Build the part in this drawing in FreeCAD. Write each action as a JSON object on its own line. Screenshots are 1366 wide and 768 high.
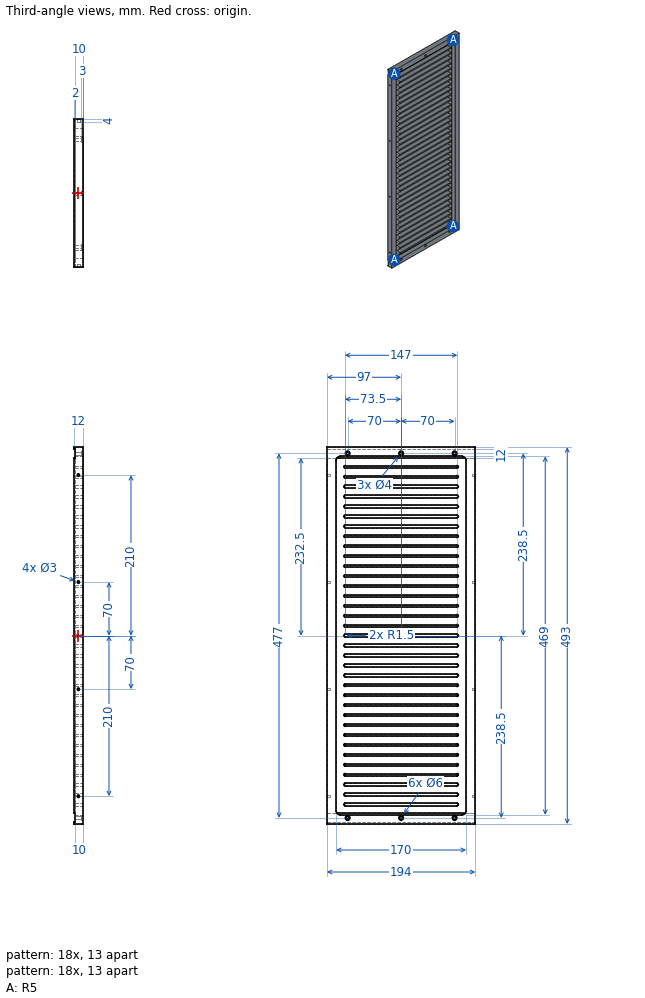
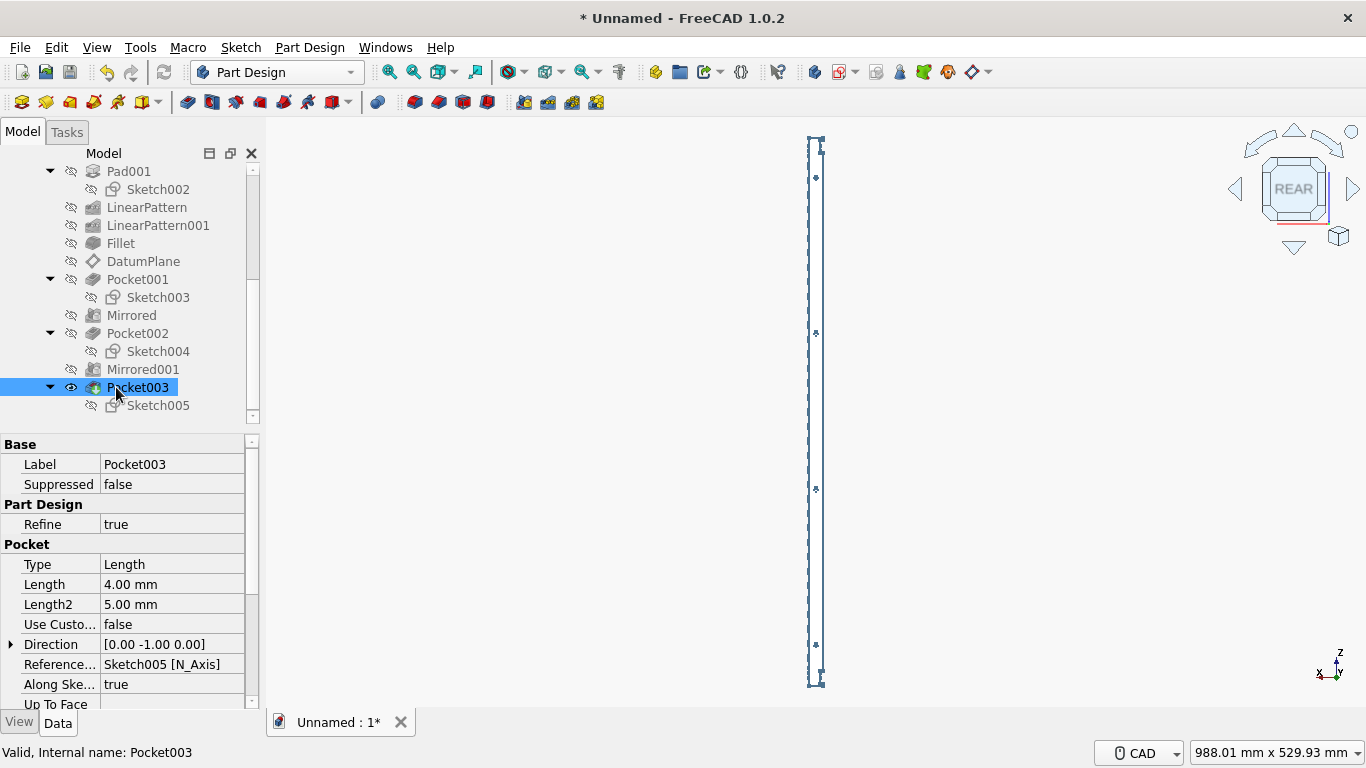
{"action": "left_click", "coordinate": [524, 102]}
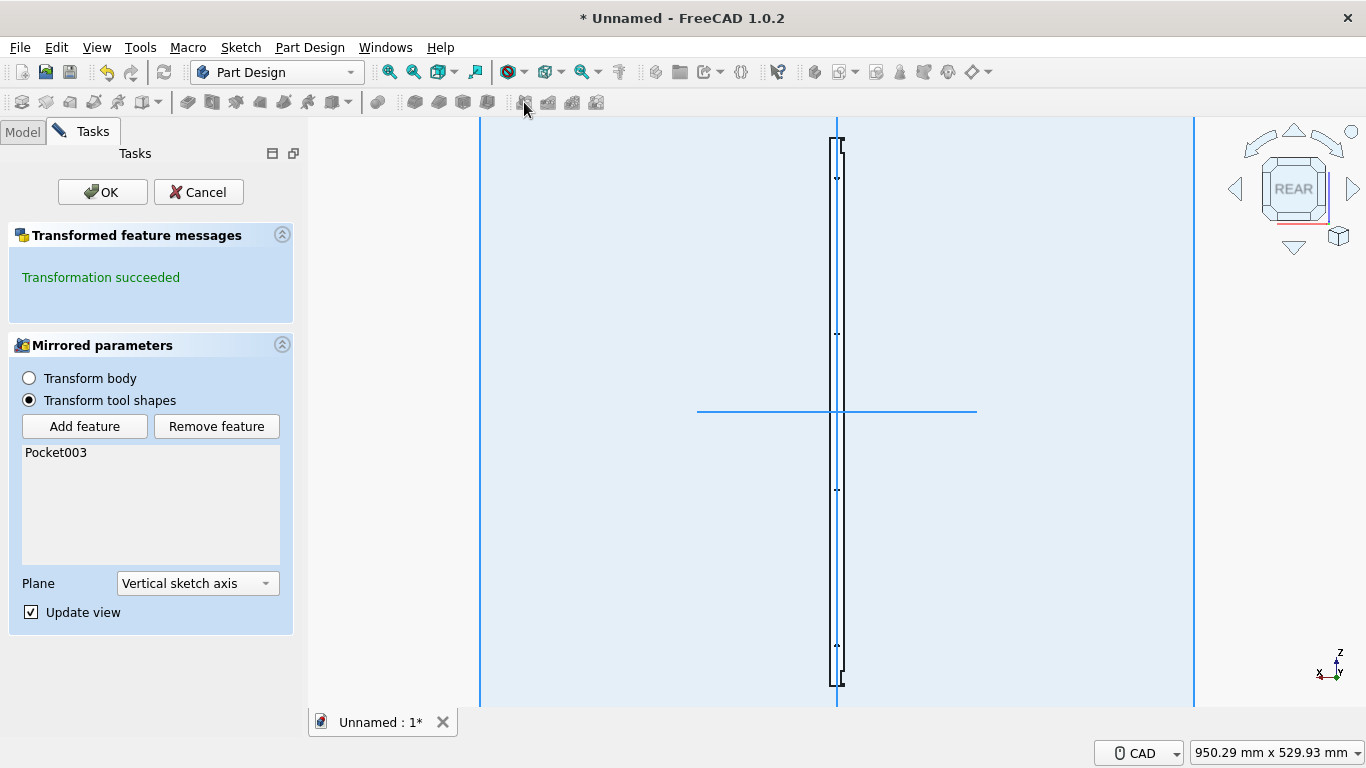
{"action": "left_click", "coordinate": [198, 584]}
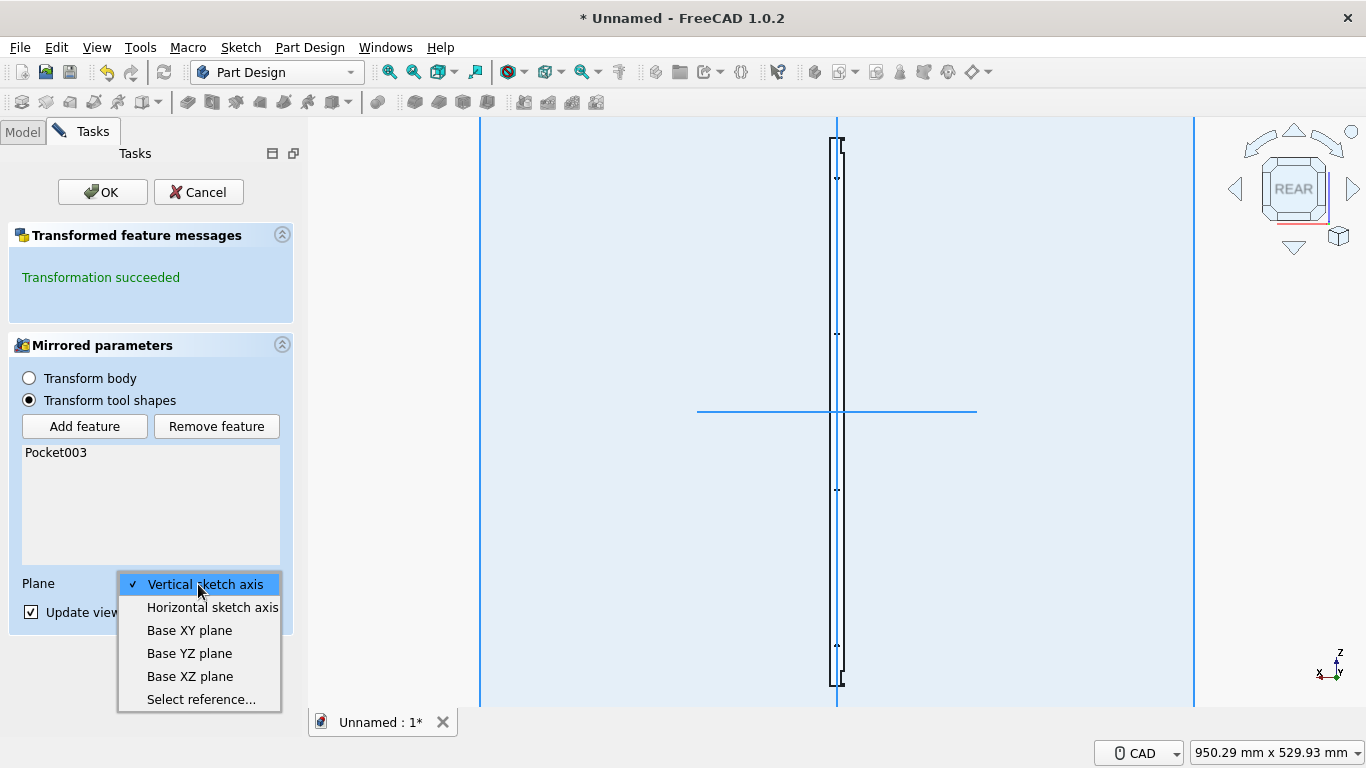
{"action": "left_click", "coordinate": [198, 676]}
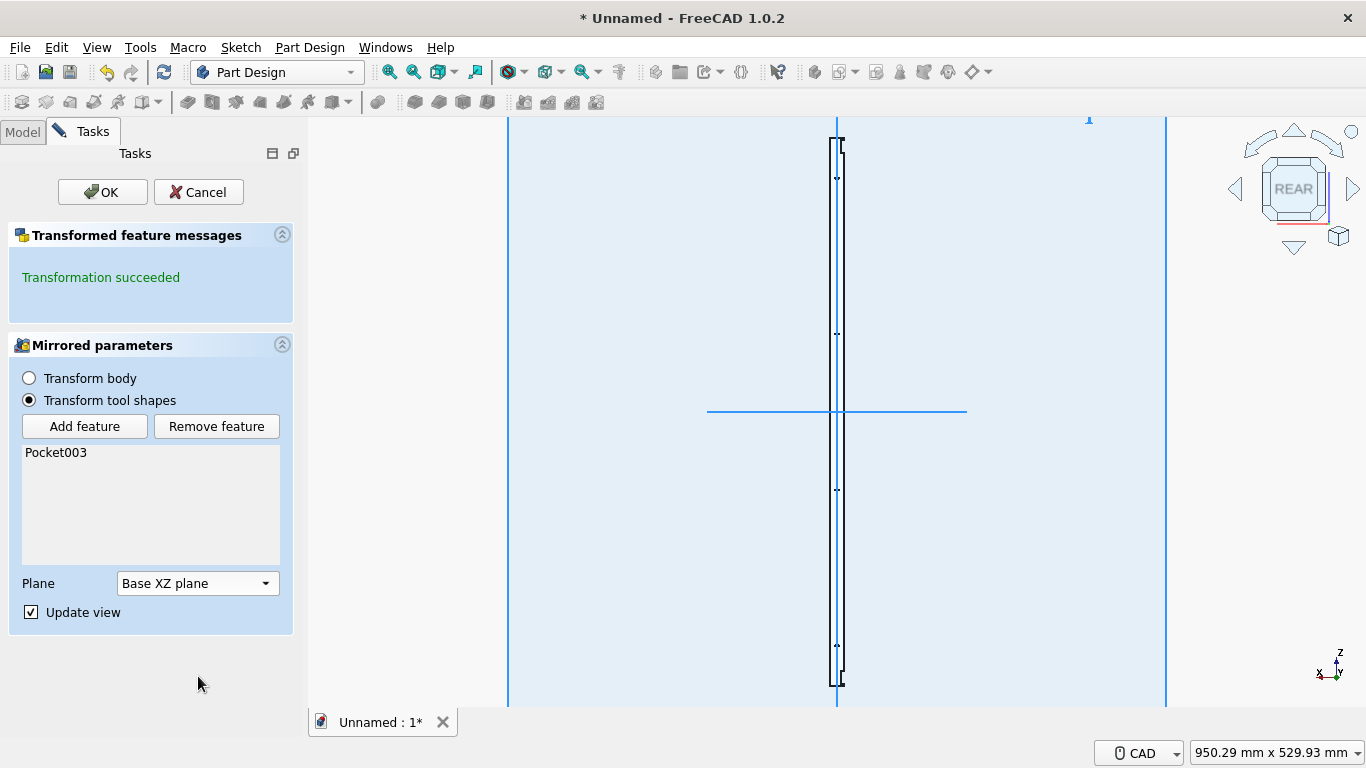
{"action": "left_click", "coordinate": [103, 192]}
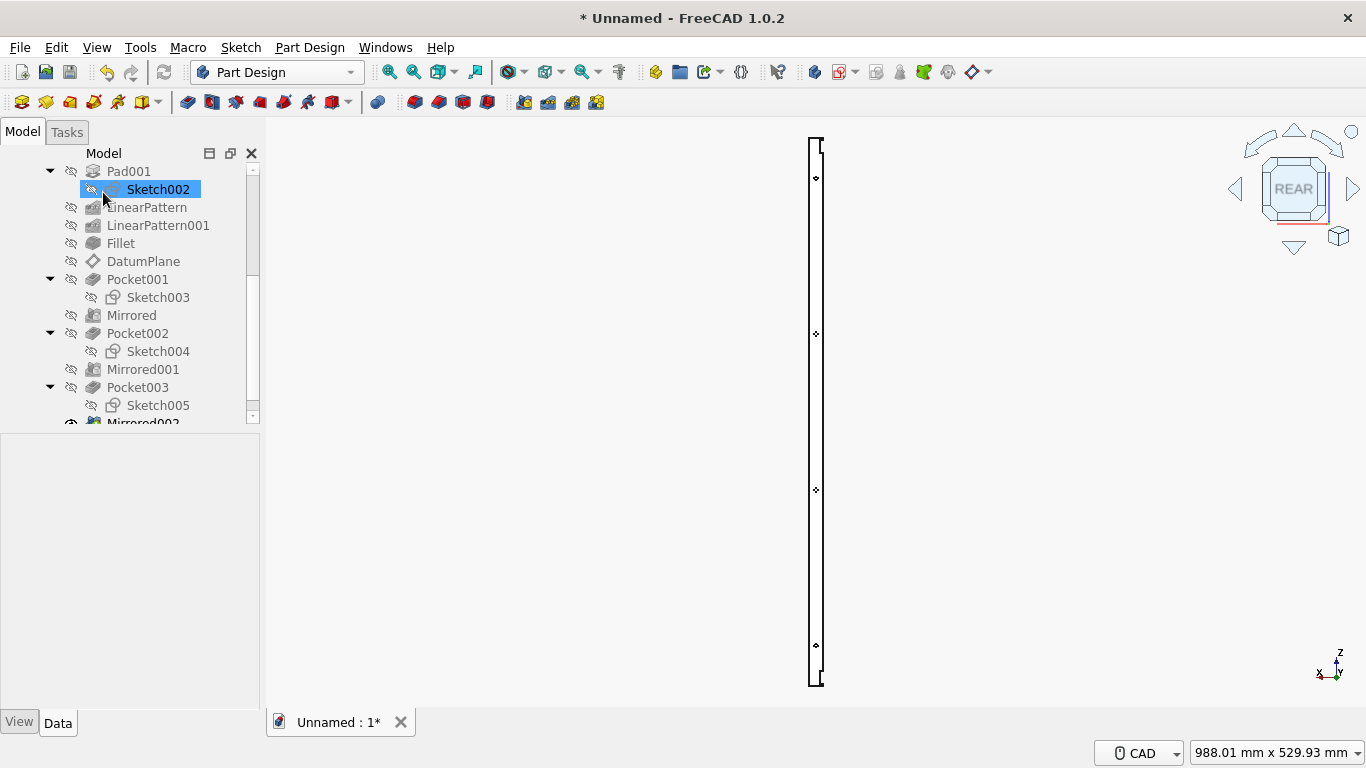
{"action": "key", "text": "0"}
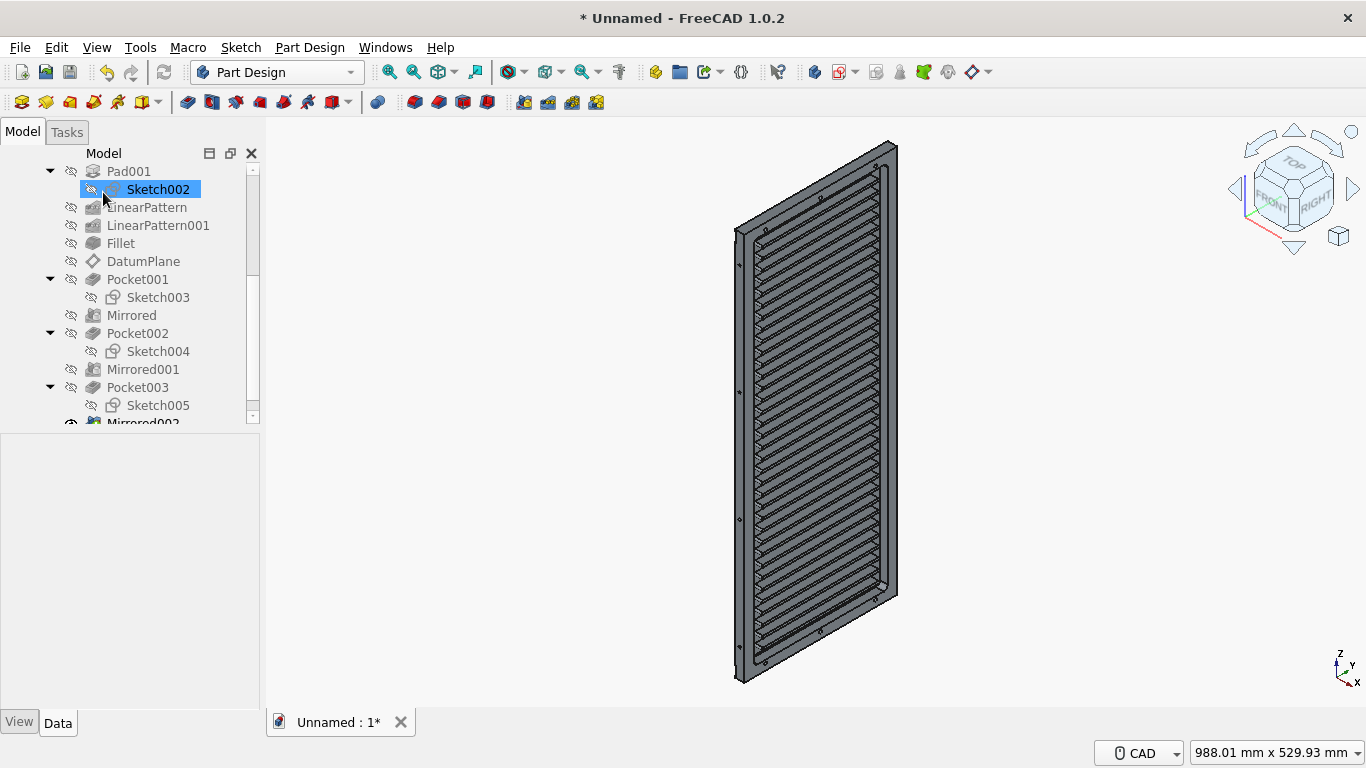
{"action": "key", "text": "3"}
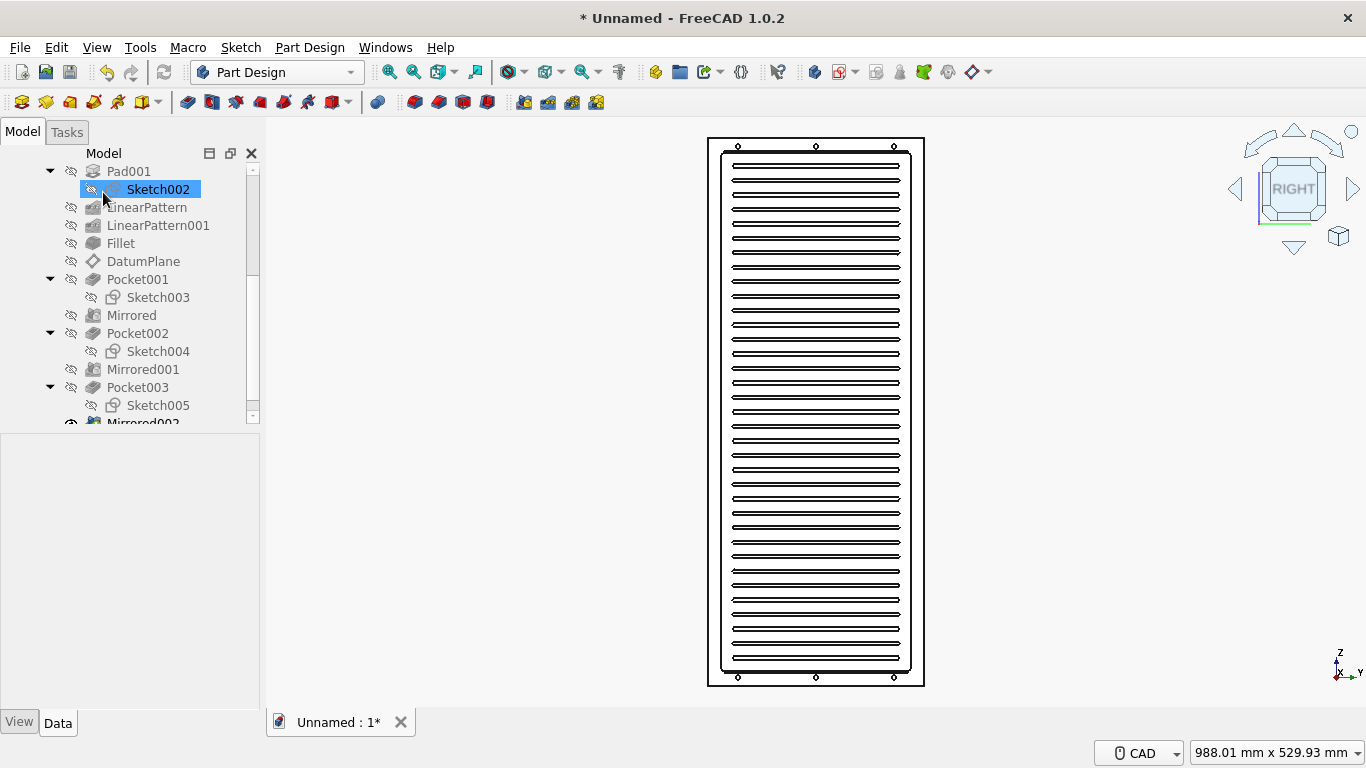
{"action": "key", "text": "2"}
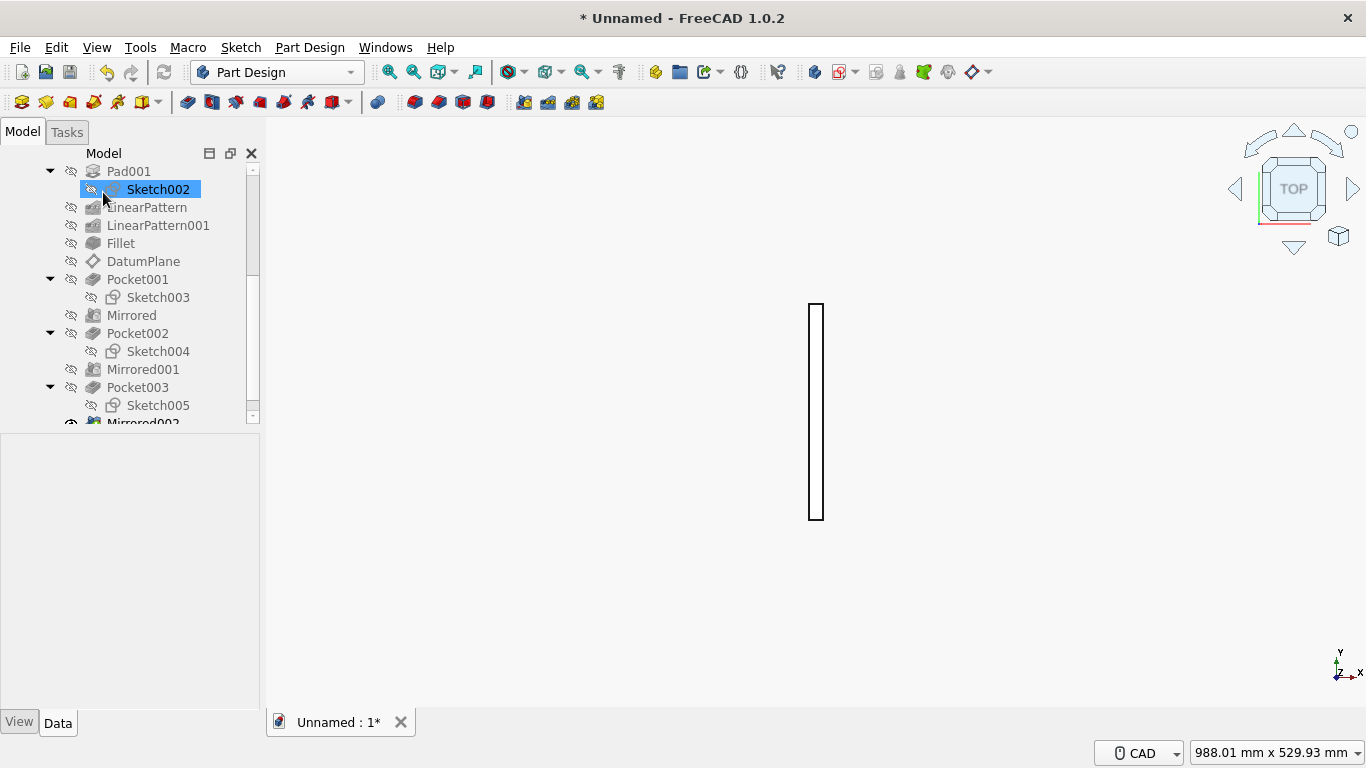
{"action": "left_click", "coordinate": [390, 72]}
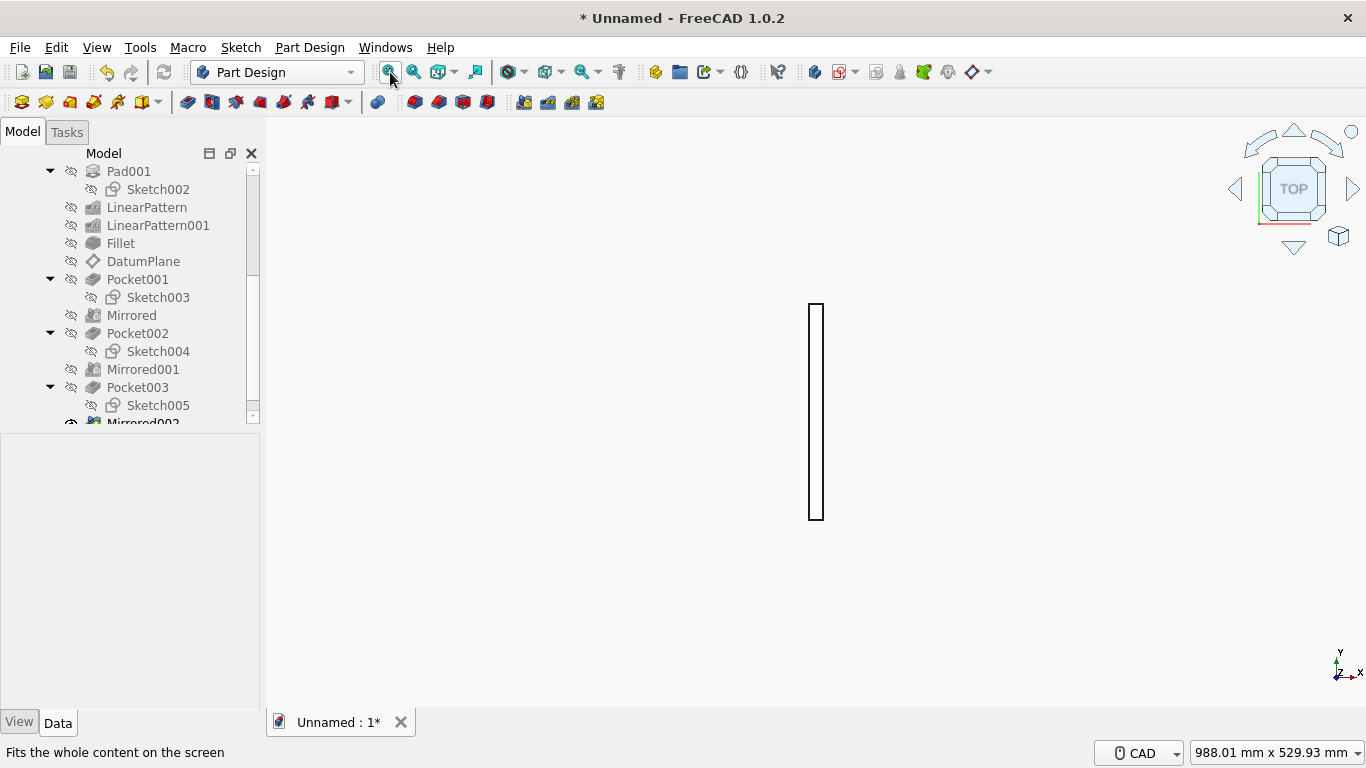
{"action": "scroll", "coordinate": [140, 293], "scroll_direction": "down", "scroll_amount": 3}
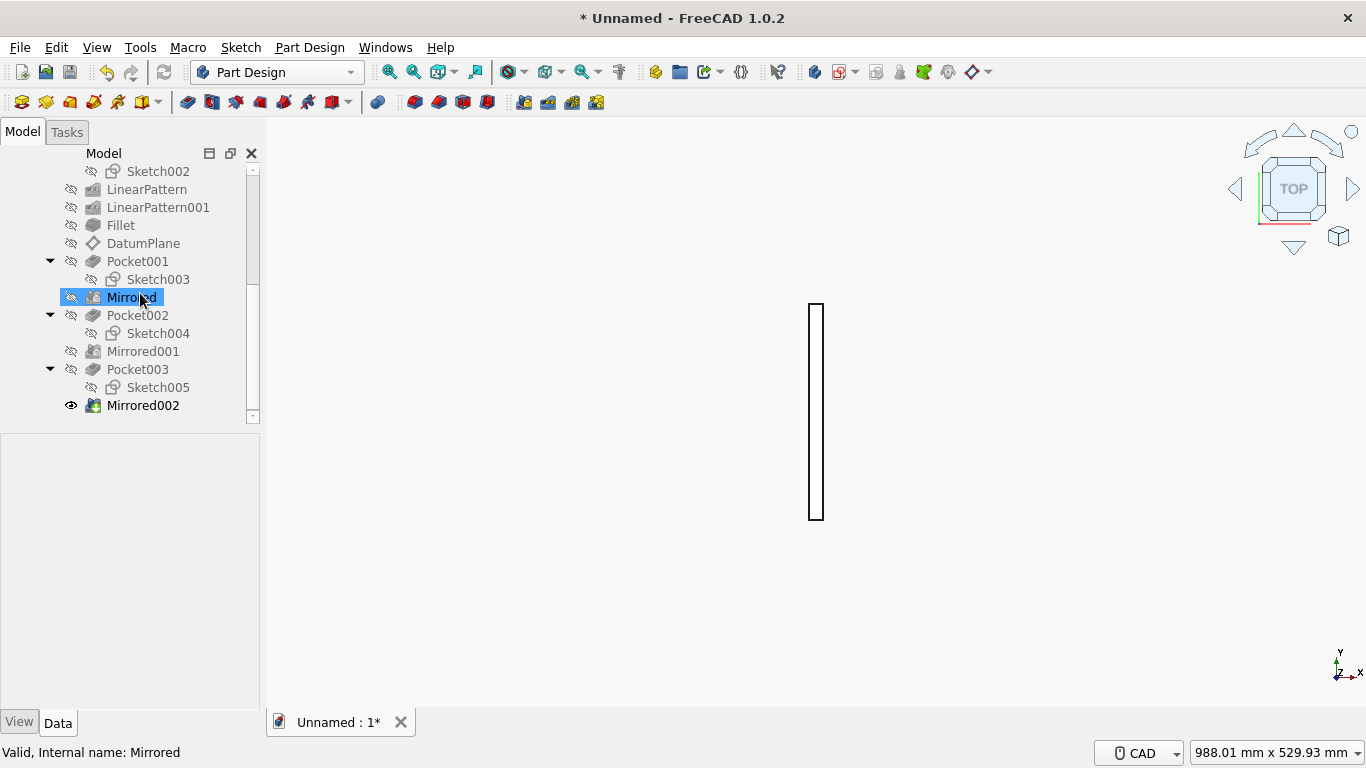
{"action": "scroll", "coordinate": [160, 293], "scroll_direction": "up", "scroll_amount": 15}